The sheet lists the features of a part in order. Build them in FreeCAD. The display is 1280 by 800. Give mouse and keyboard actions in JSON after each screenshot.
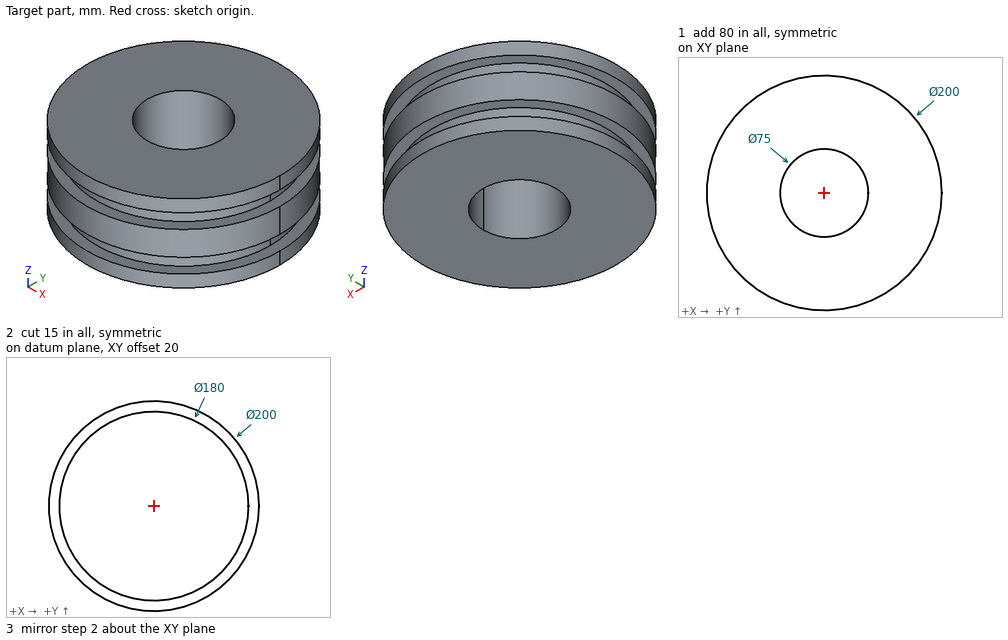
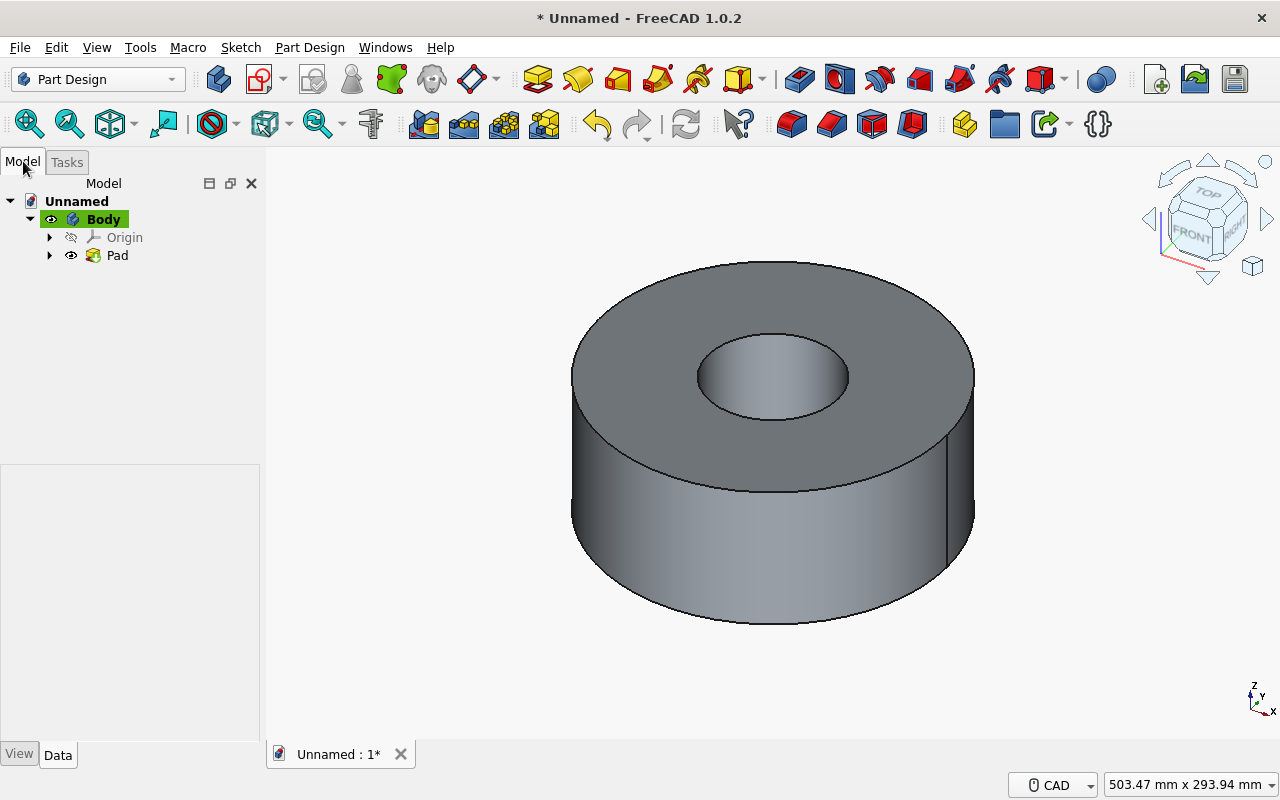
{"action": "left_click", "coordinate": [50, 237]}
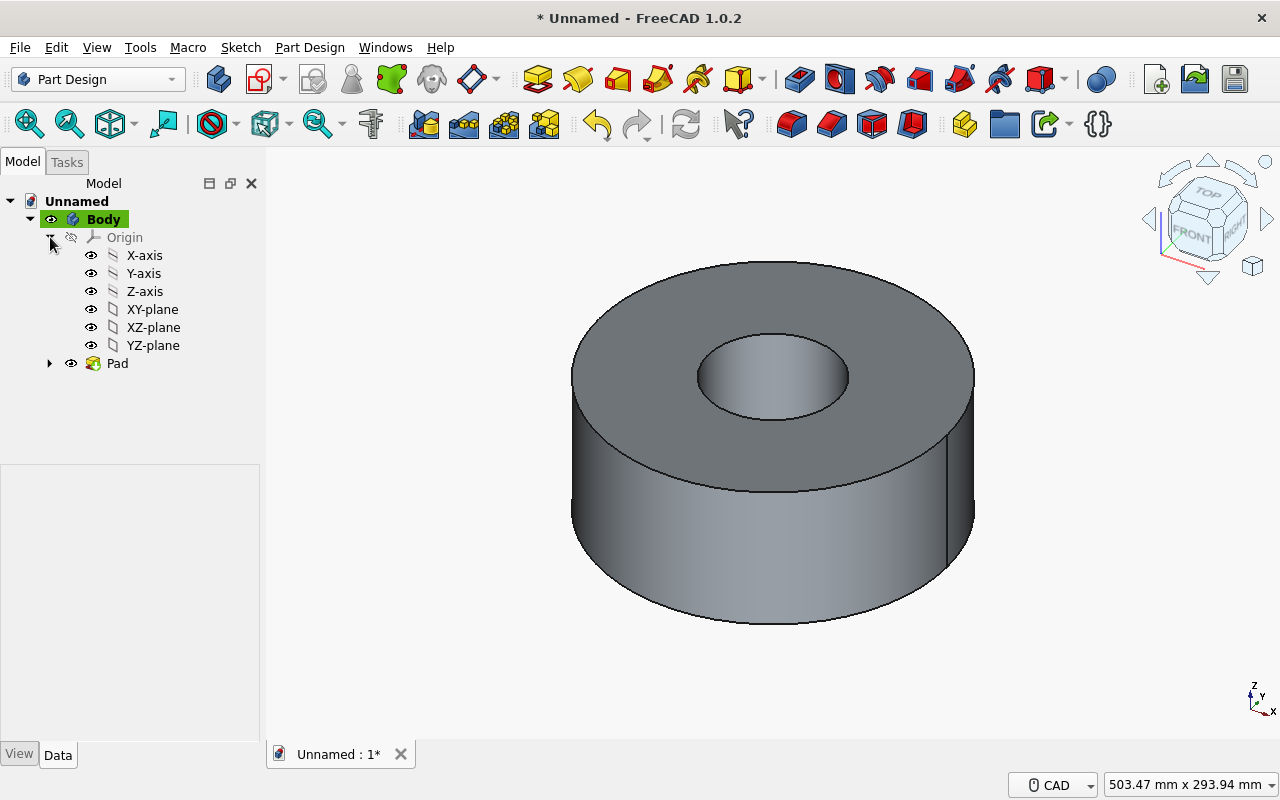
{"action": "left_click", "coordinate": [136, 309]}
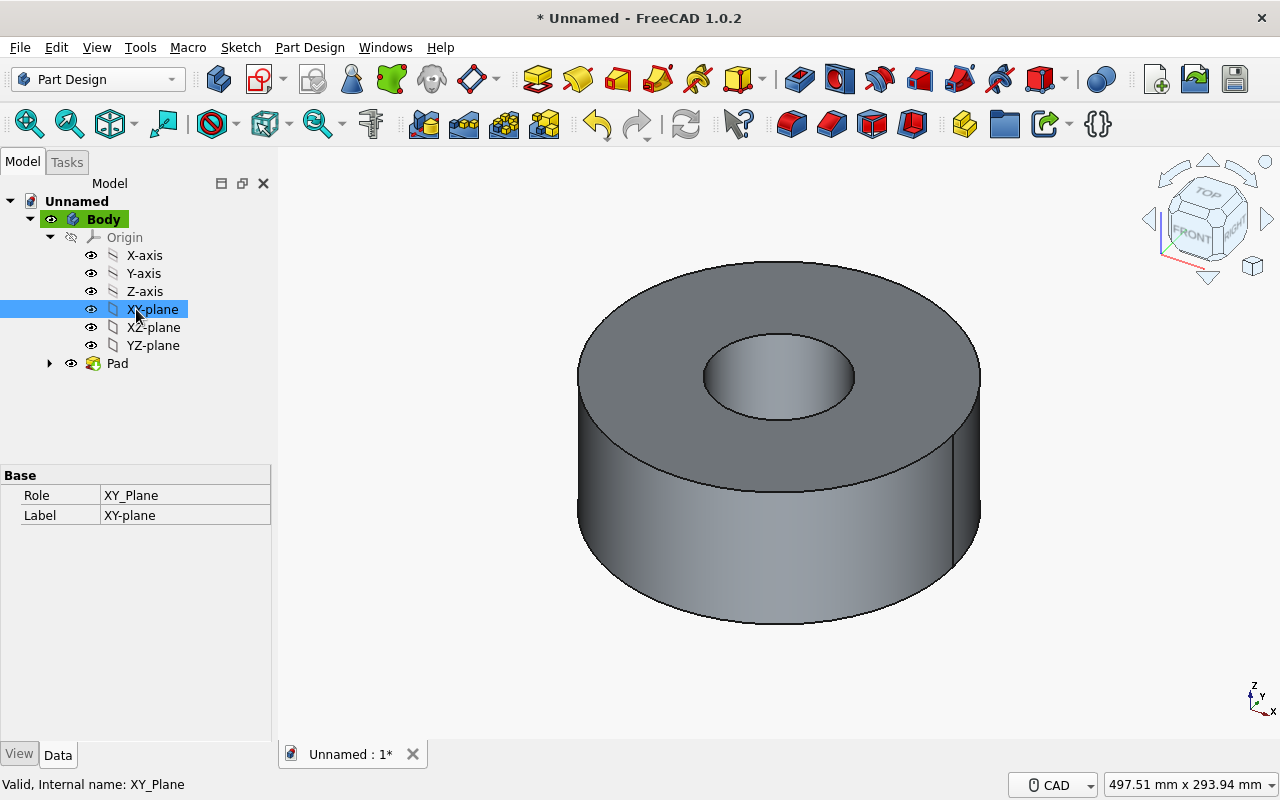
{"action": "left_click", "coordinate": [472, 80]}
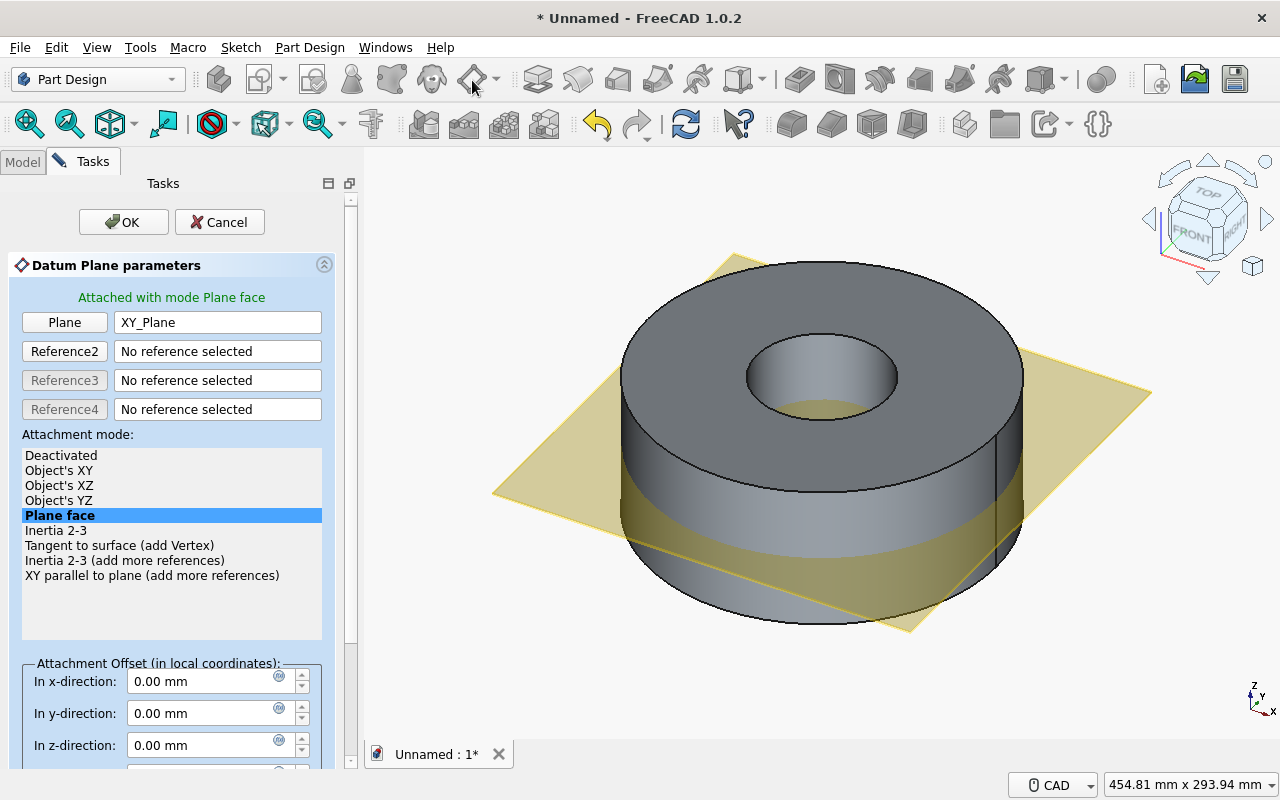
{"action": "triple_click", "coordinate": [210, 745]}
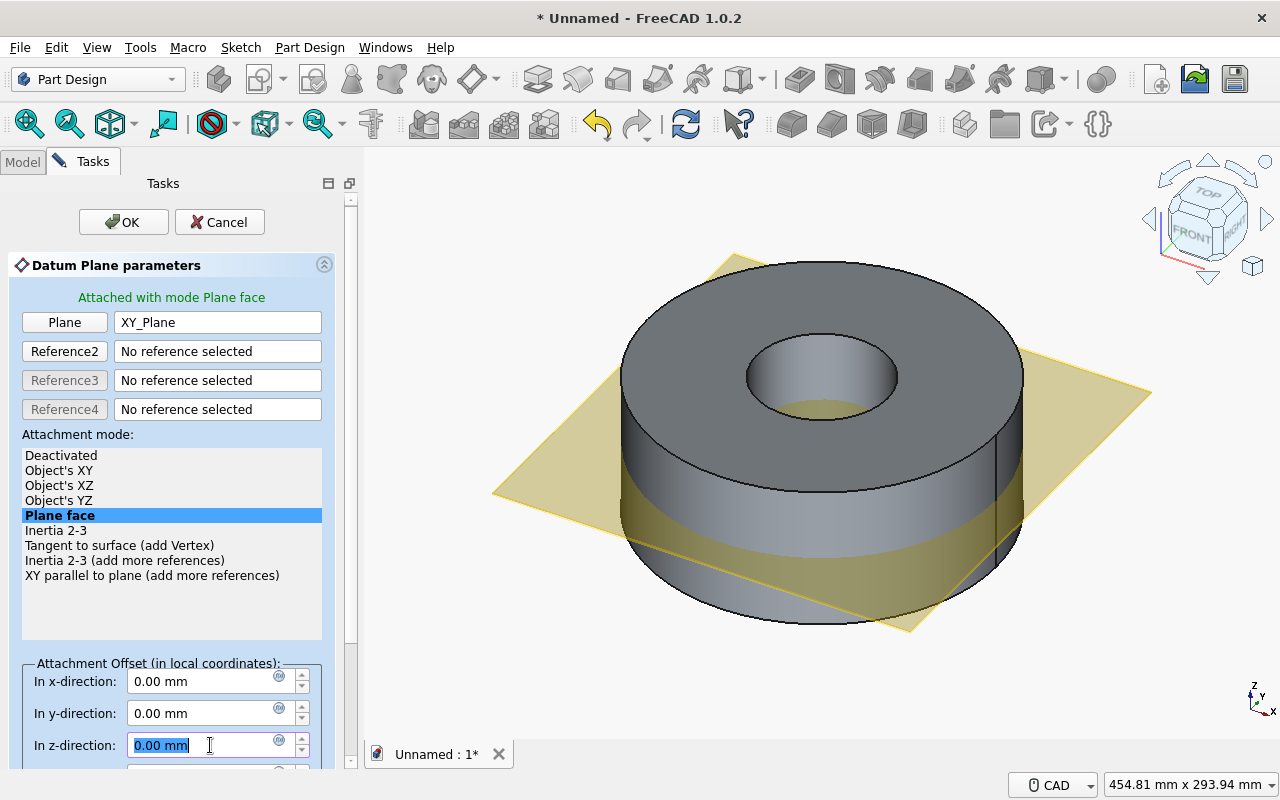
{"action": "type", "text": "20"}
{"action": "key", "text": "Tab"}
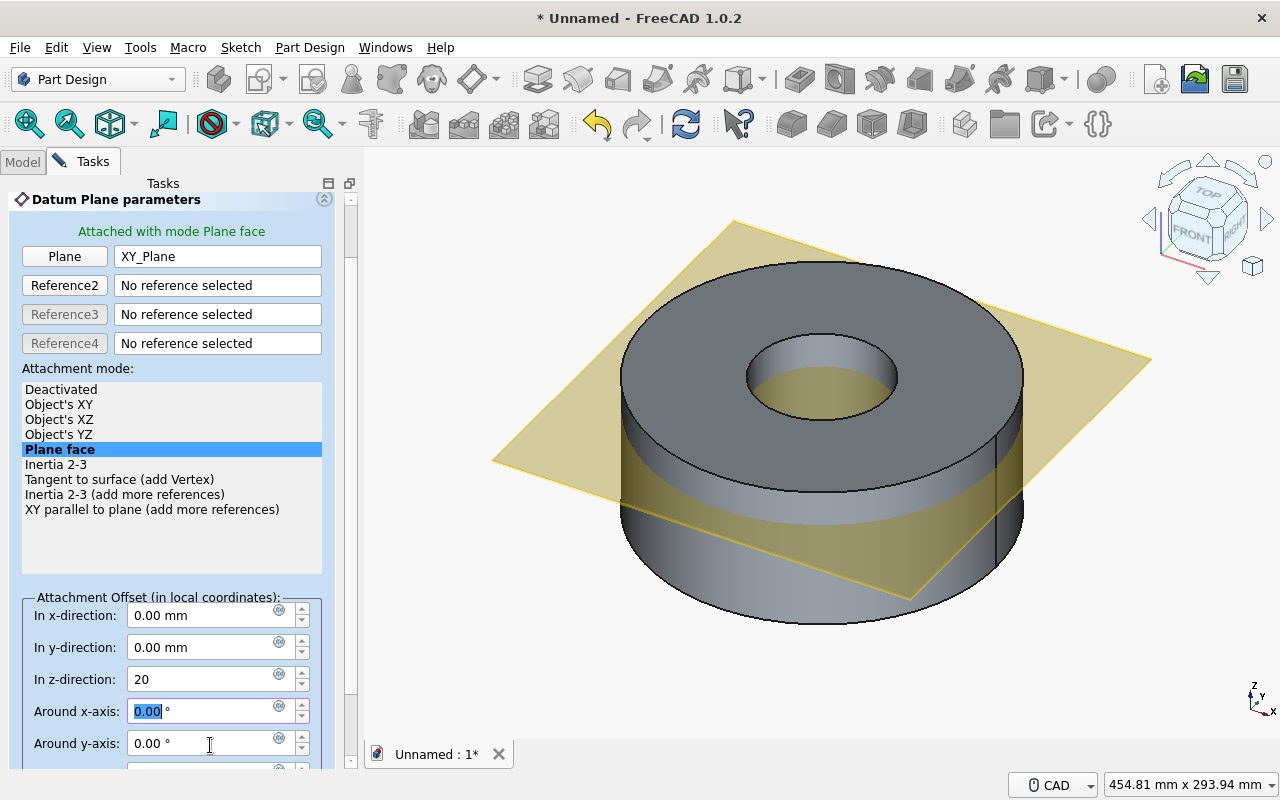
{"action": "scroll", "coordinate": [351, 480], "scroll_direction": "up", "scroll_amount": 2}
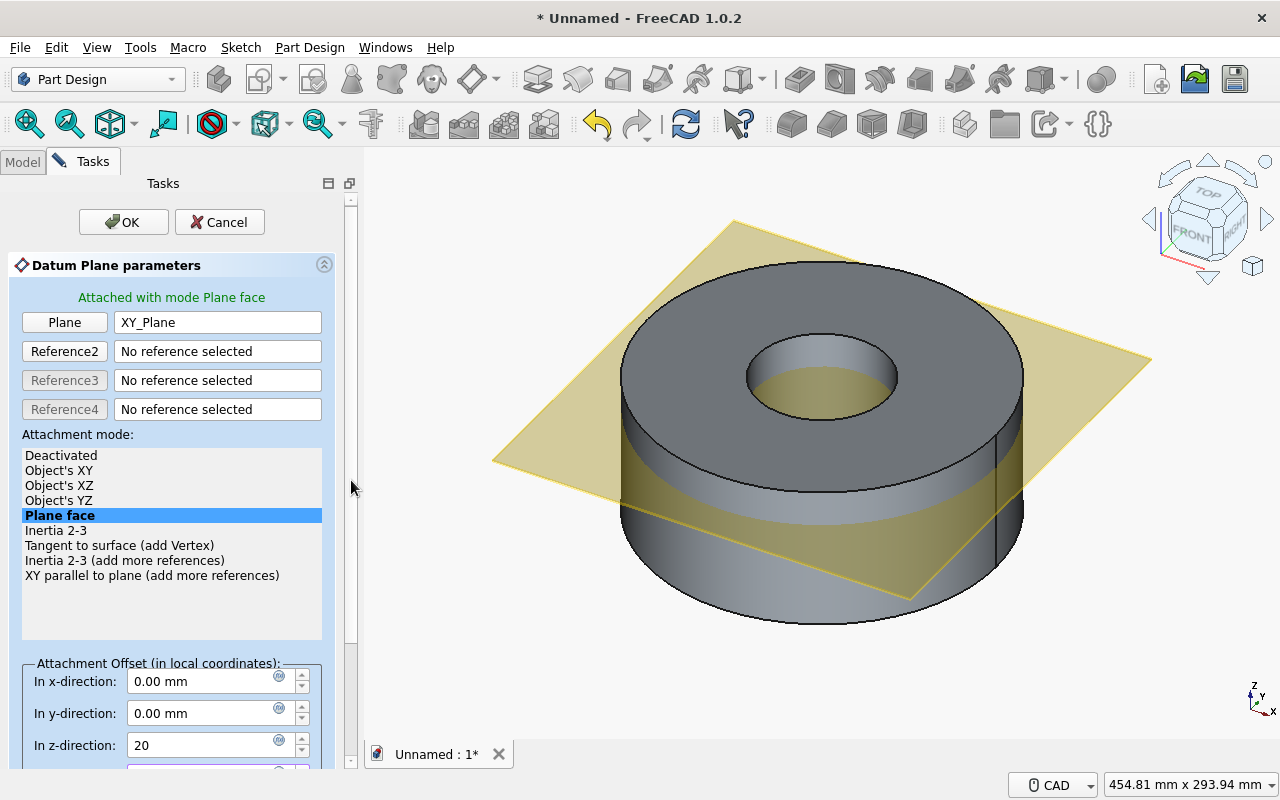
{"action": "left_click", "coordinate": [124, 222]}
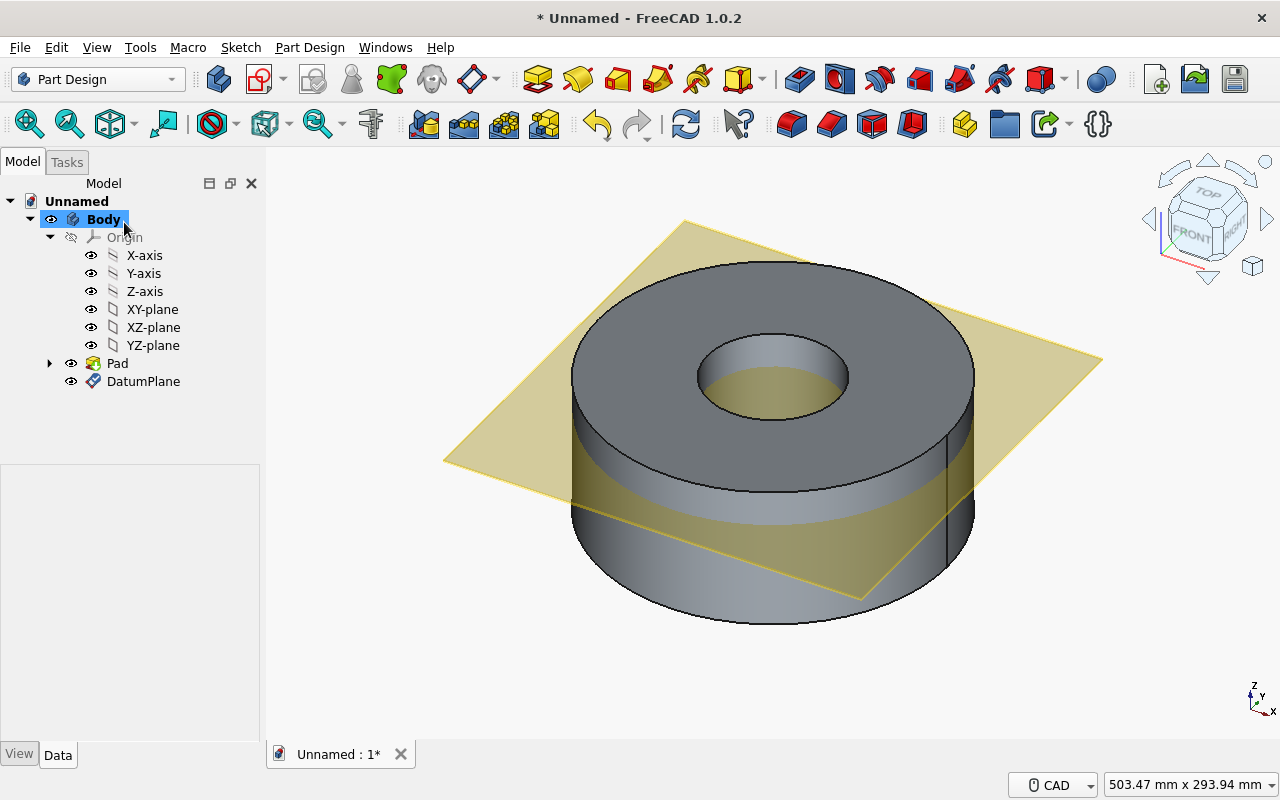
{"action": "left_click", "coordinate": [116, 381]}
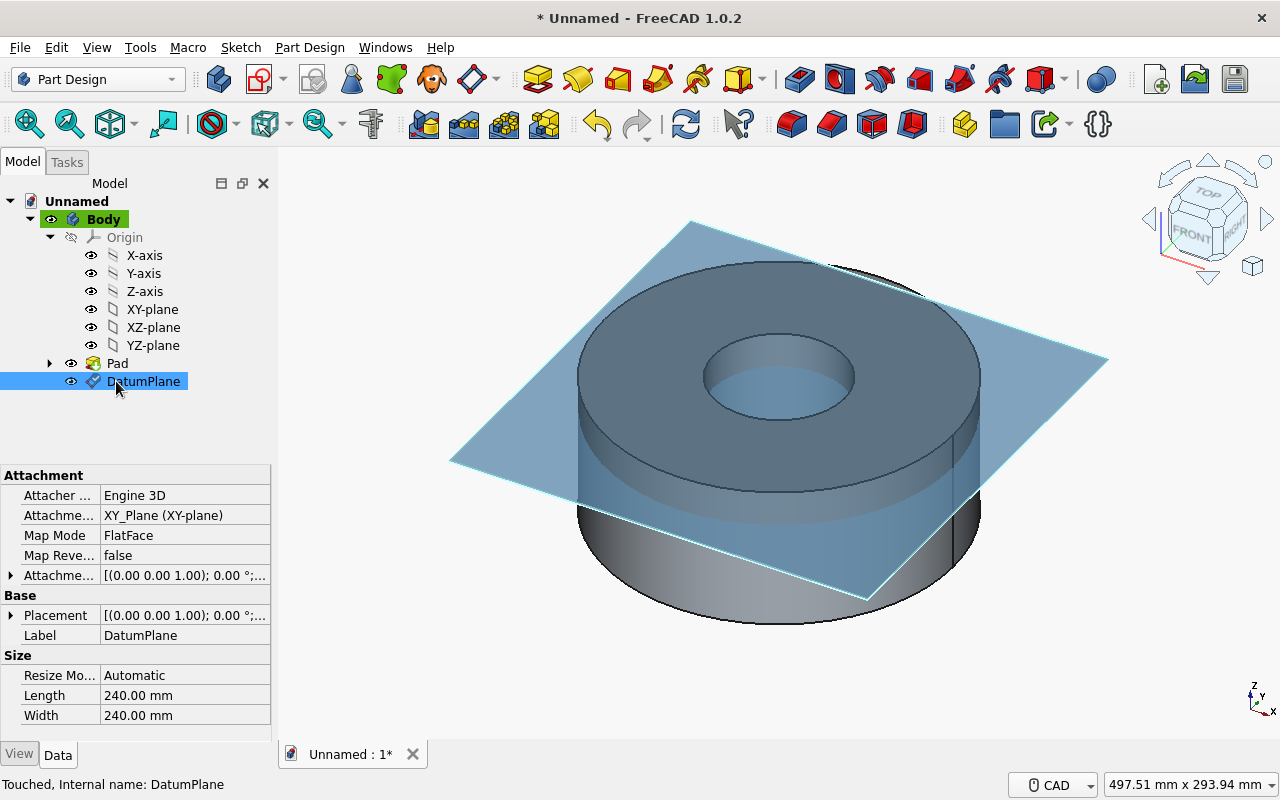
{"action": "left_click", "coordinate": [260, 80]}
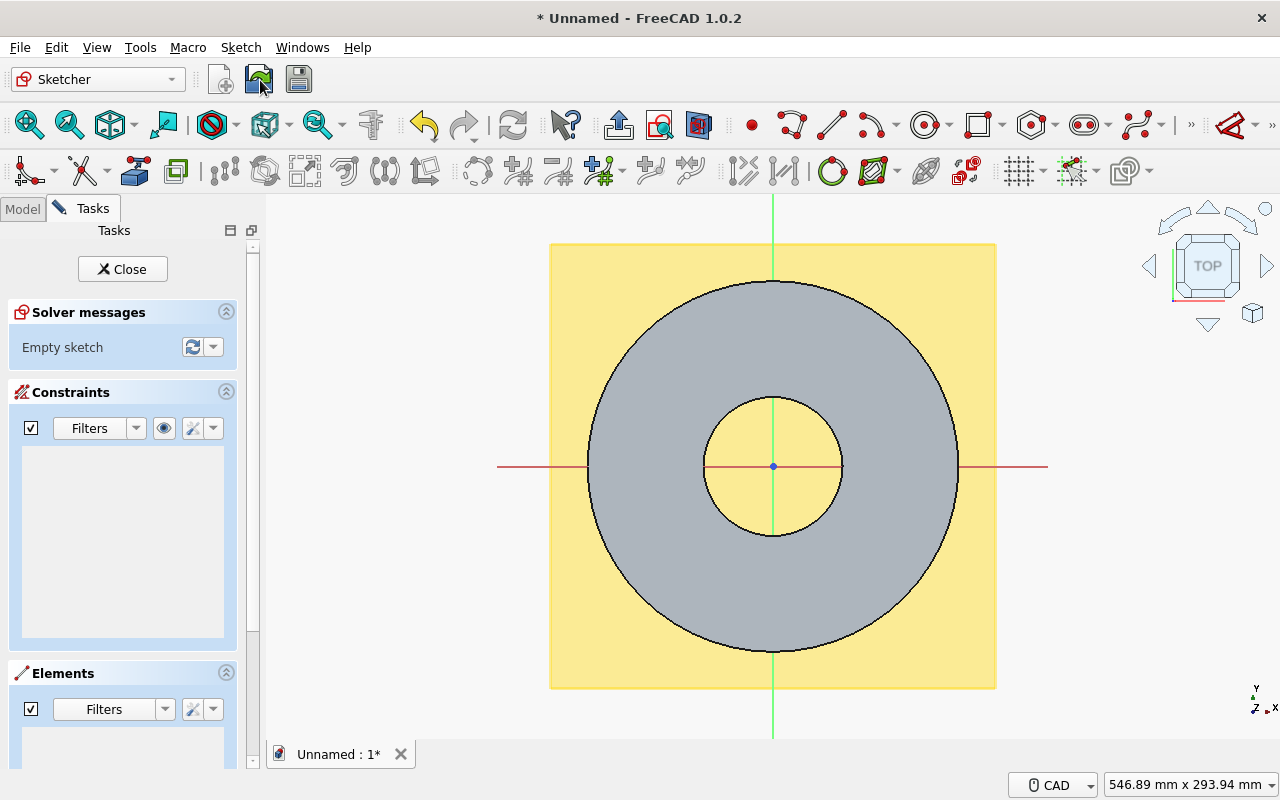
{"action": "left_click", "coordinate": [700, 126]}